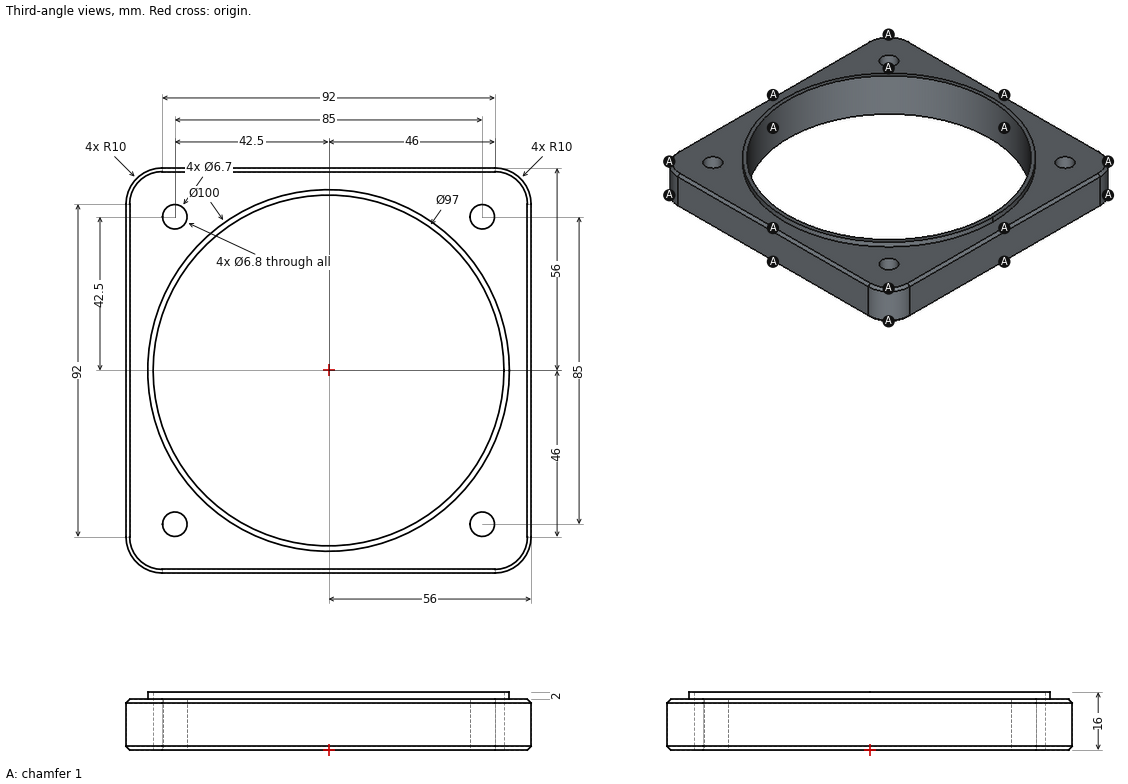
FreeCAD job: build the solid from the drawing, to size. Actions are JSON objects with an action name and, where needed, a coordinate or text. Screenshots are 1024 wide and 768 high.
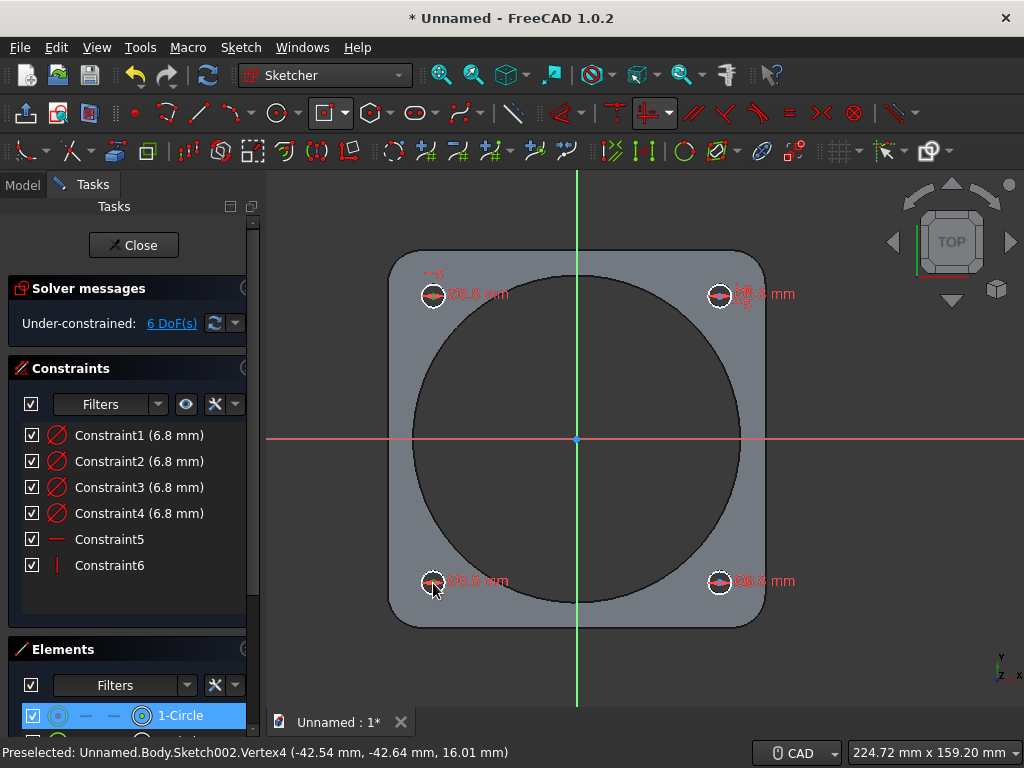
{"action": "left_click", "coordinate": [672, 114]}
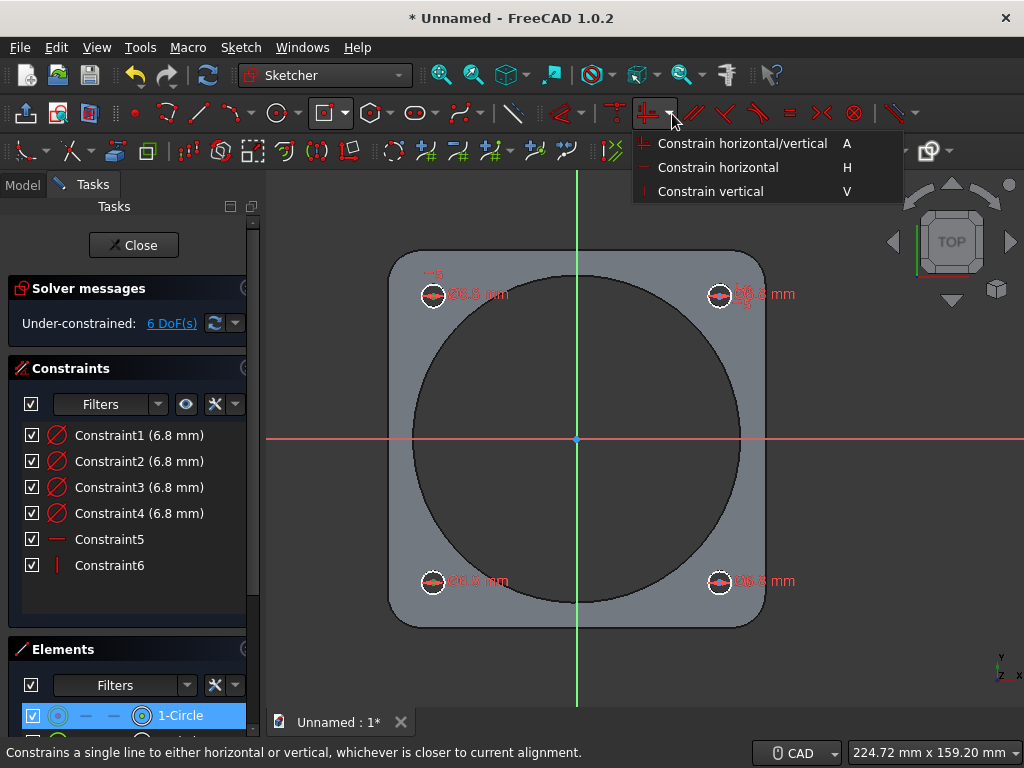
{"action": "left_click", "coordinate": [768, 191]}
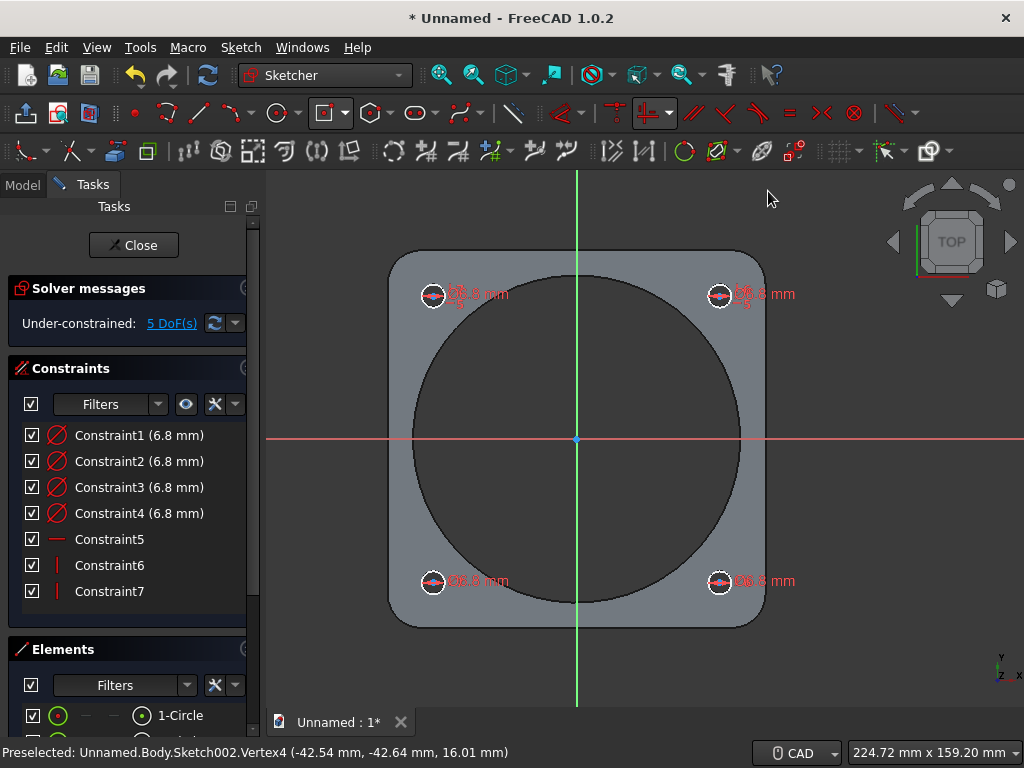
{"action": "left_click", "coordinate": [720, 583]}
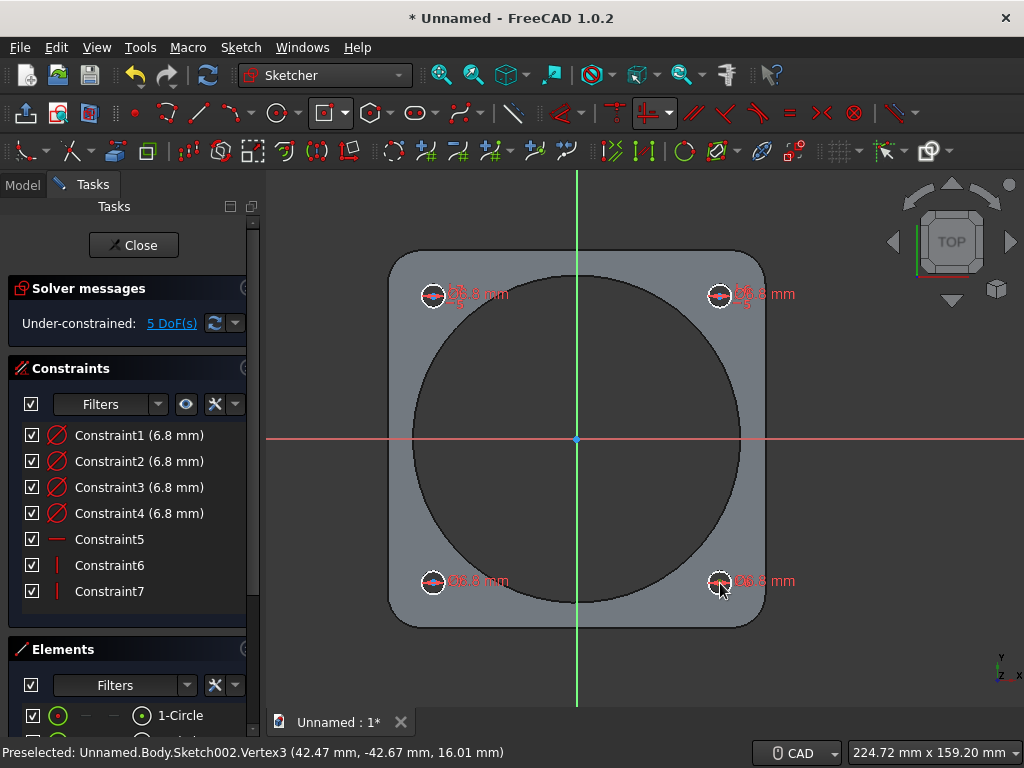
{"action": "left_click", "coordinate": [433, 583]}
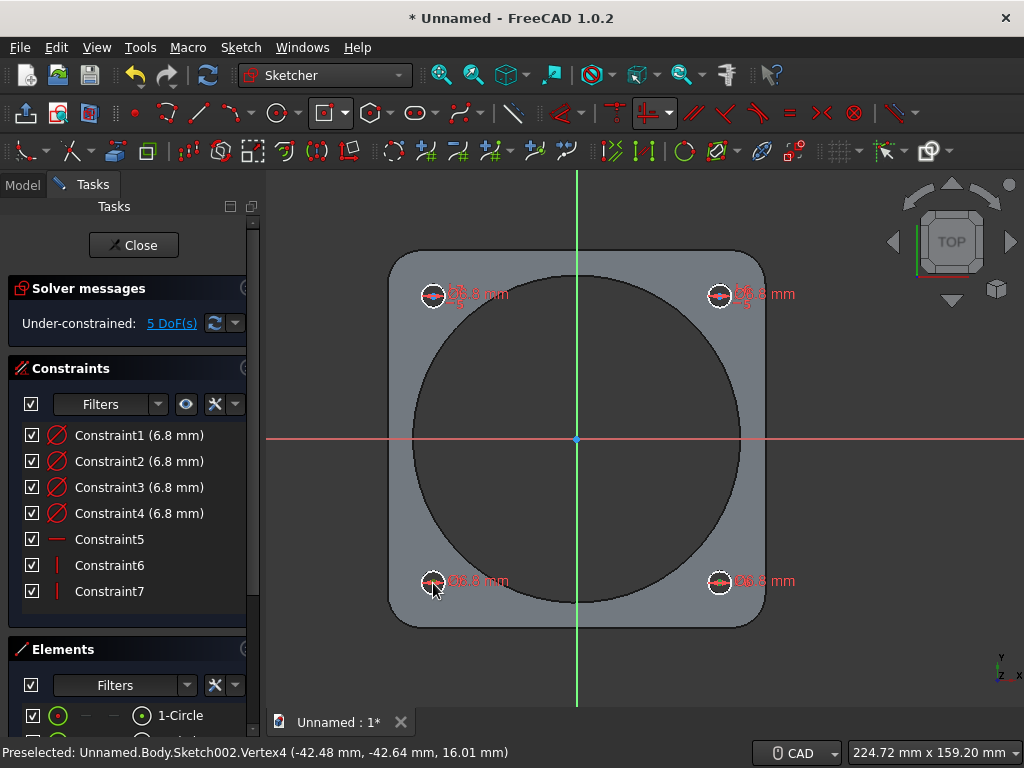
{"action": "left_click", "coordinate": [672, 114]}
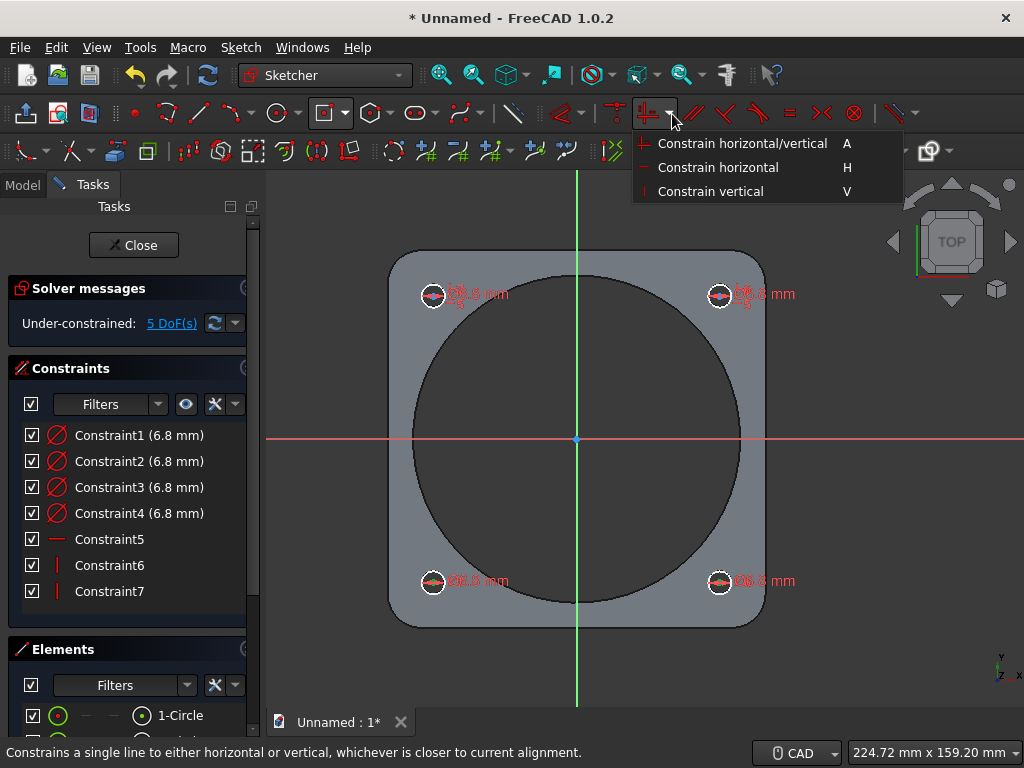
{"action": "left_click", "coordinate": [768, 167]}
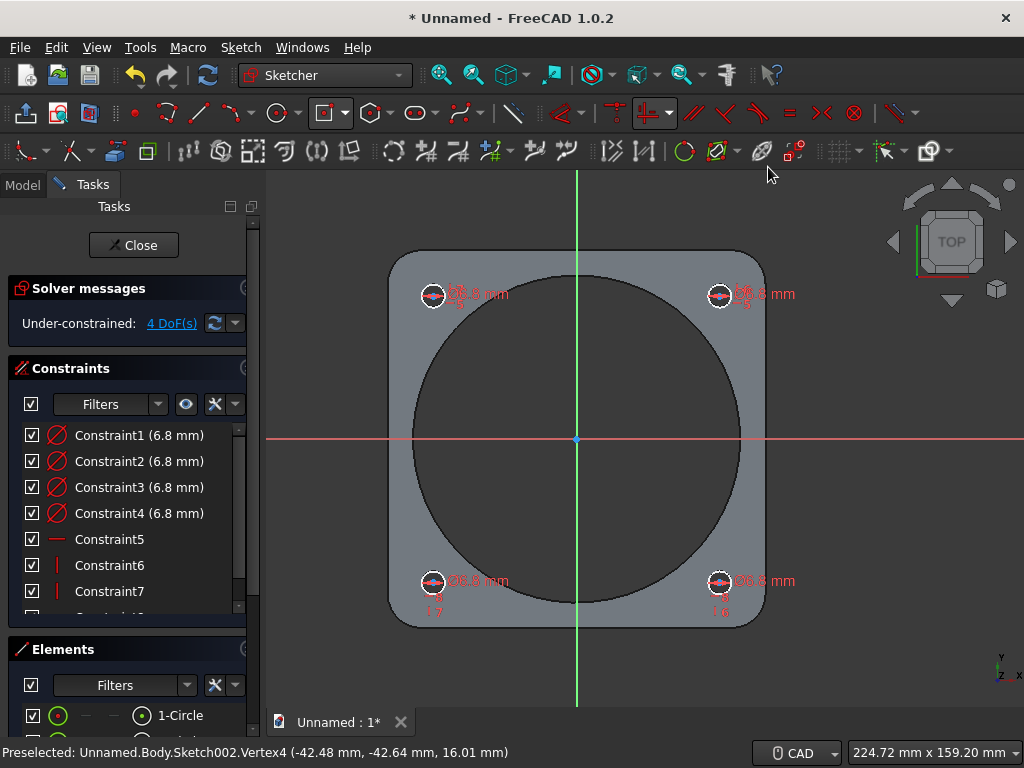
{"action": "left_click", "coordinate": [560, 114]}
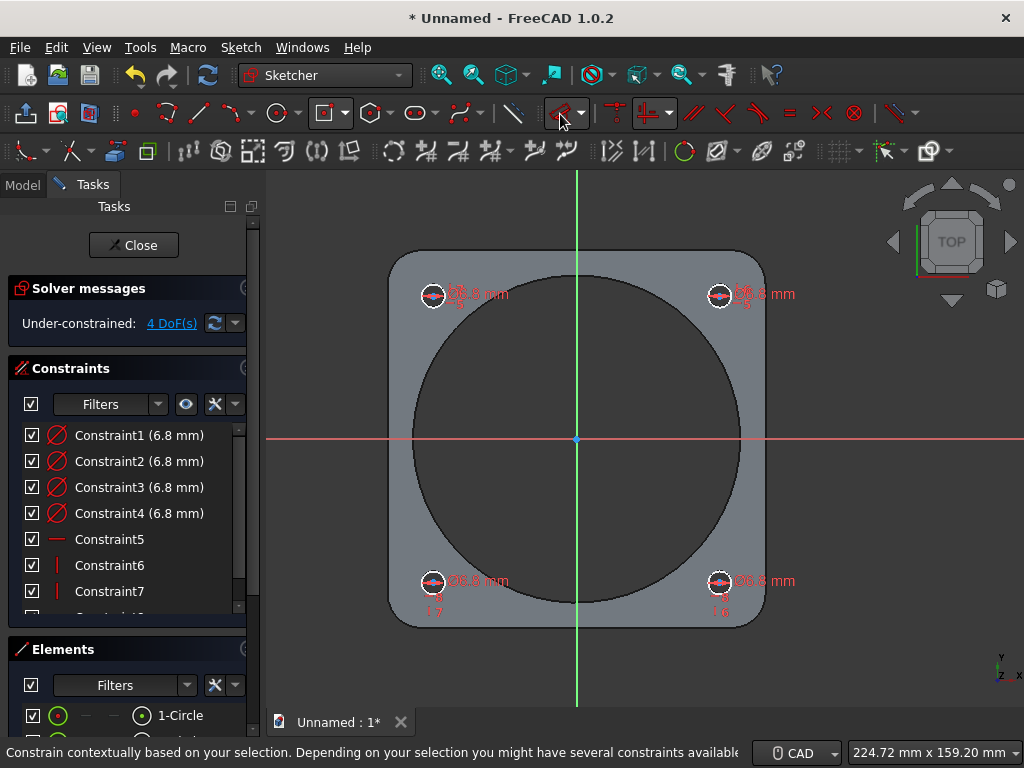
{"action": "left_click", "coordinate": [433, 296]}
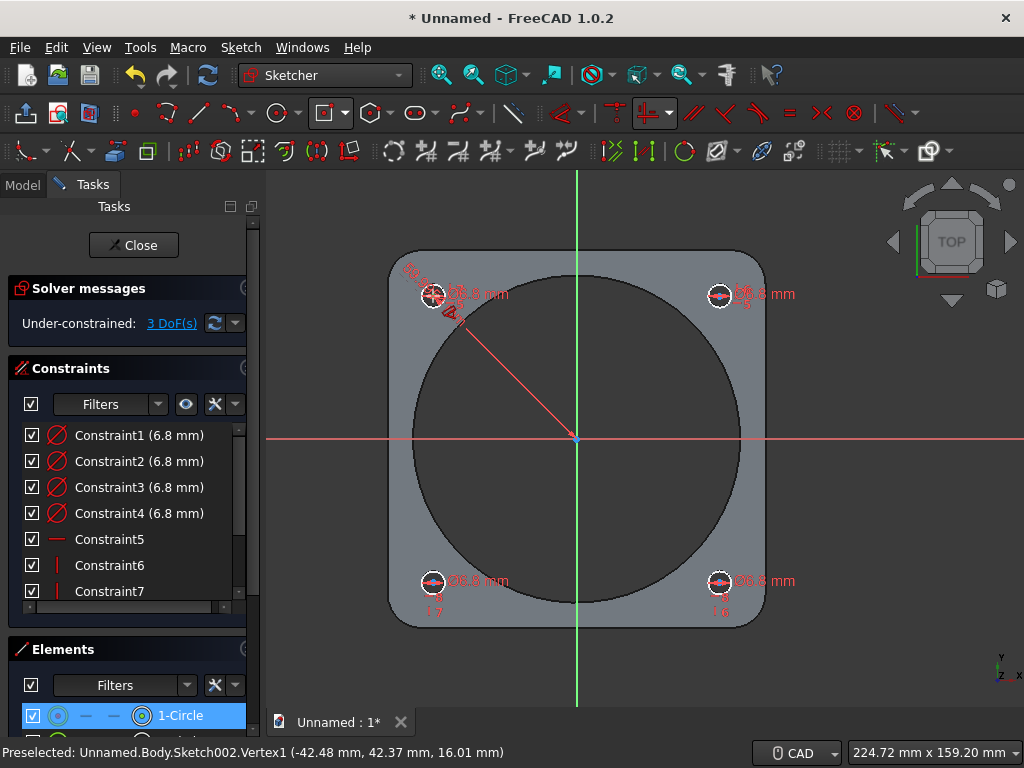
{"action": "left_click", "coordinate": [720, 296]}
{"action": "left_click", "coordinate": [511, 262]}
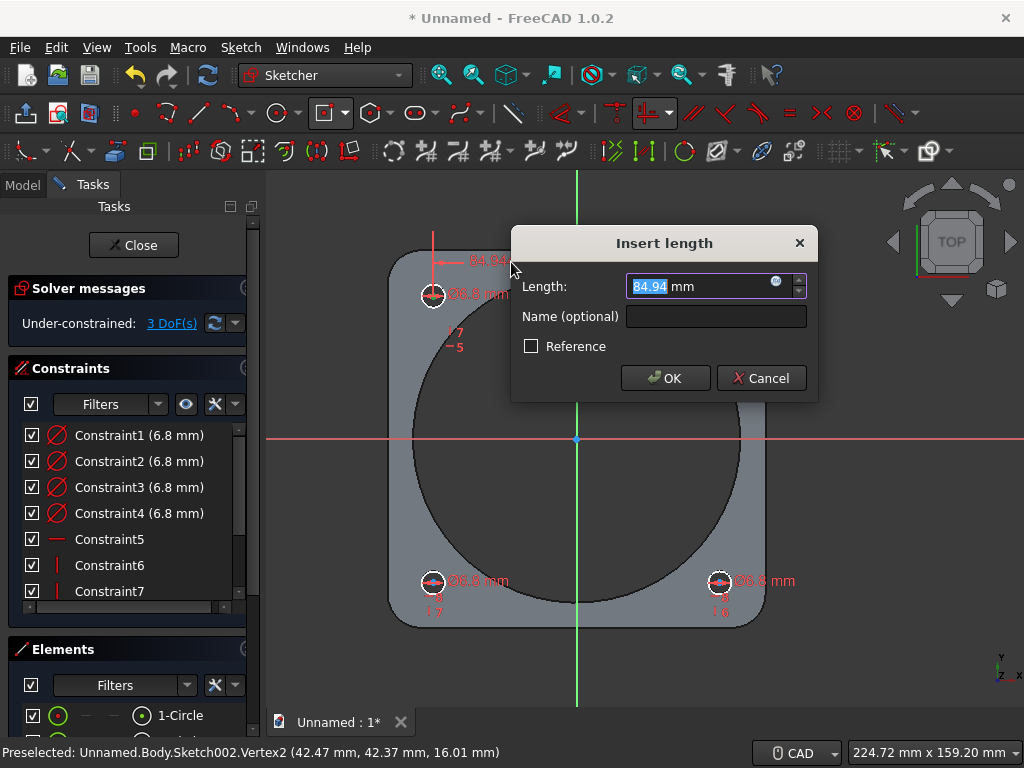
{"action": "type", "text": "85"}
{"action": "key", "text": "Return"}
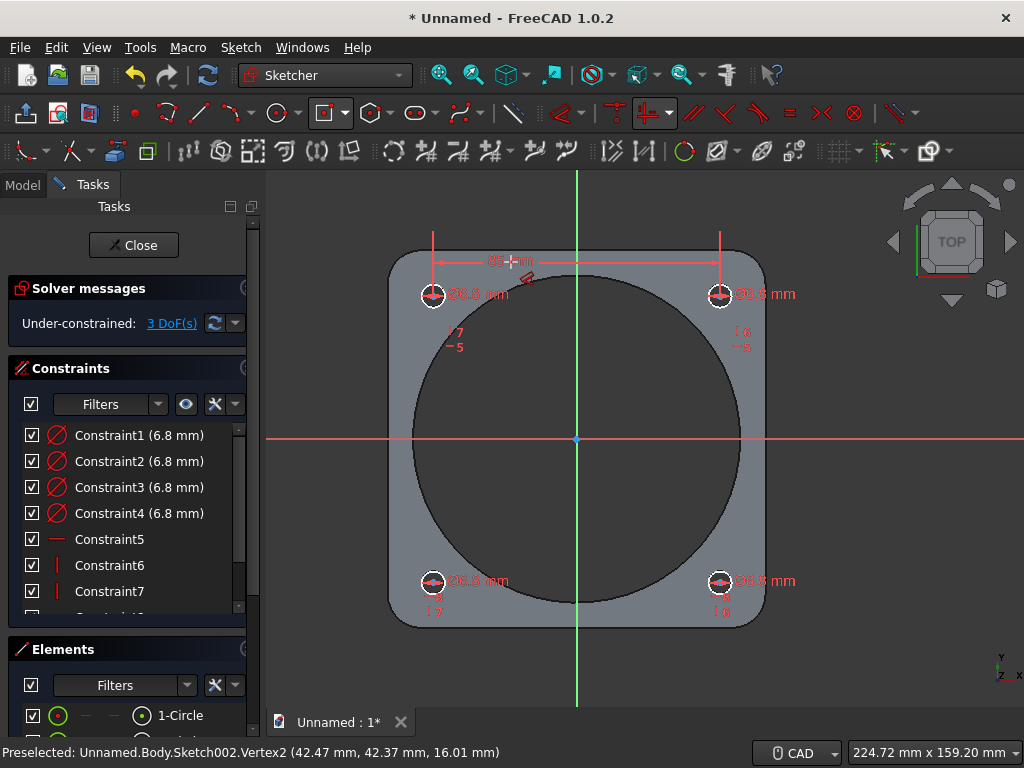
{"action": "left_click", "coordinate": [720, 296]}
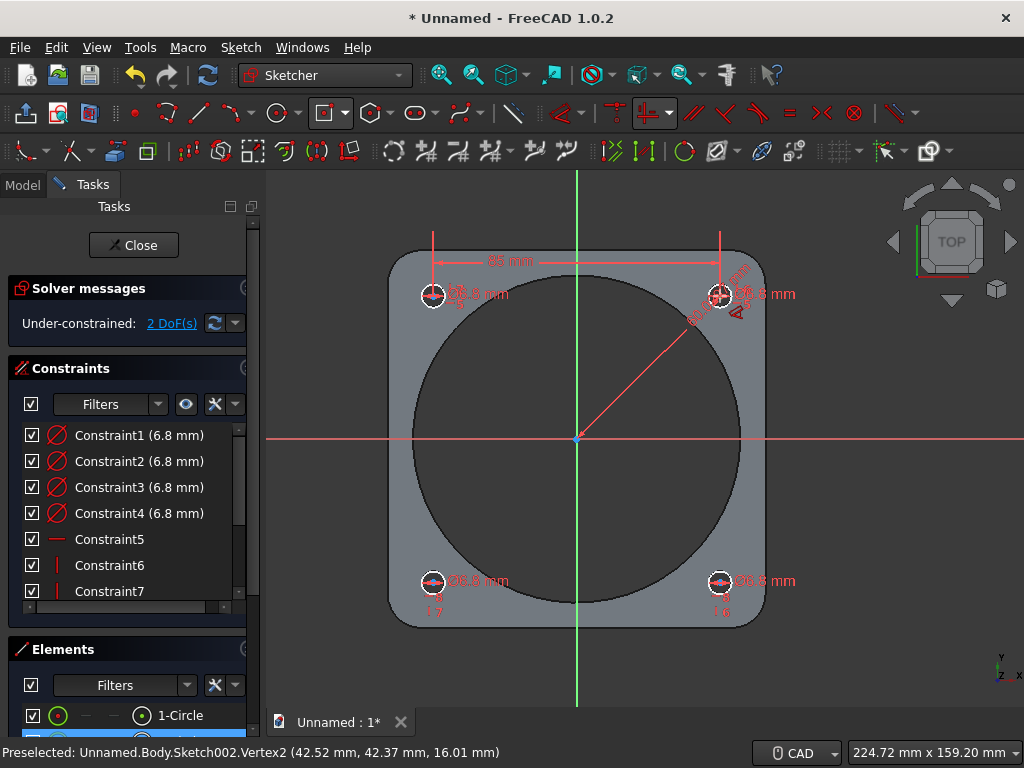
{"action": "left_click", "coordinate": [720, 583]}
{"action": "left_click", "coordinate": [754, 374]}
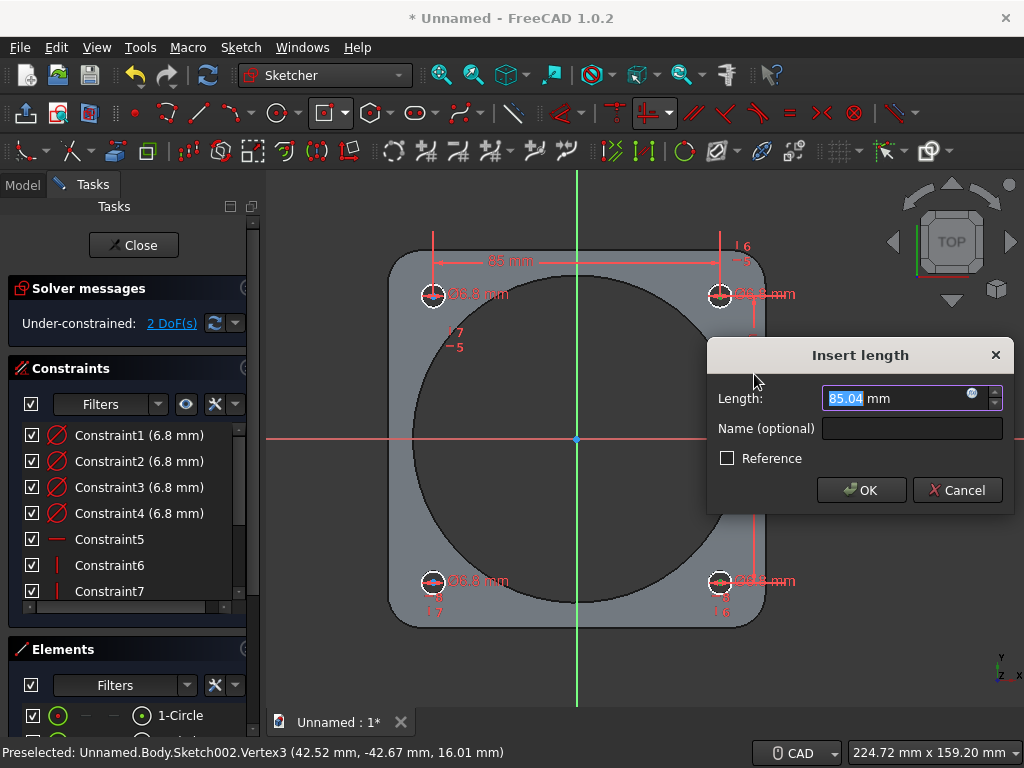
{"action": "type", "text": "85"}
{"action": "key", "text": "Return"}